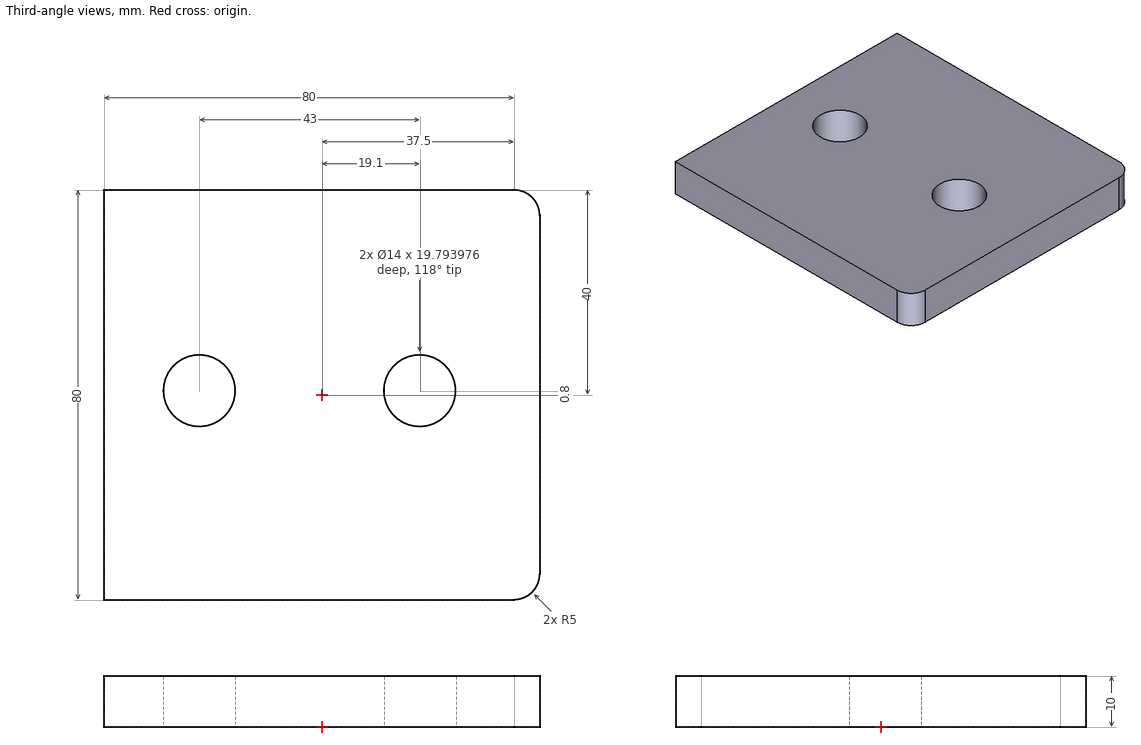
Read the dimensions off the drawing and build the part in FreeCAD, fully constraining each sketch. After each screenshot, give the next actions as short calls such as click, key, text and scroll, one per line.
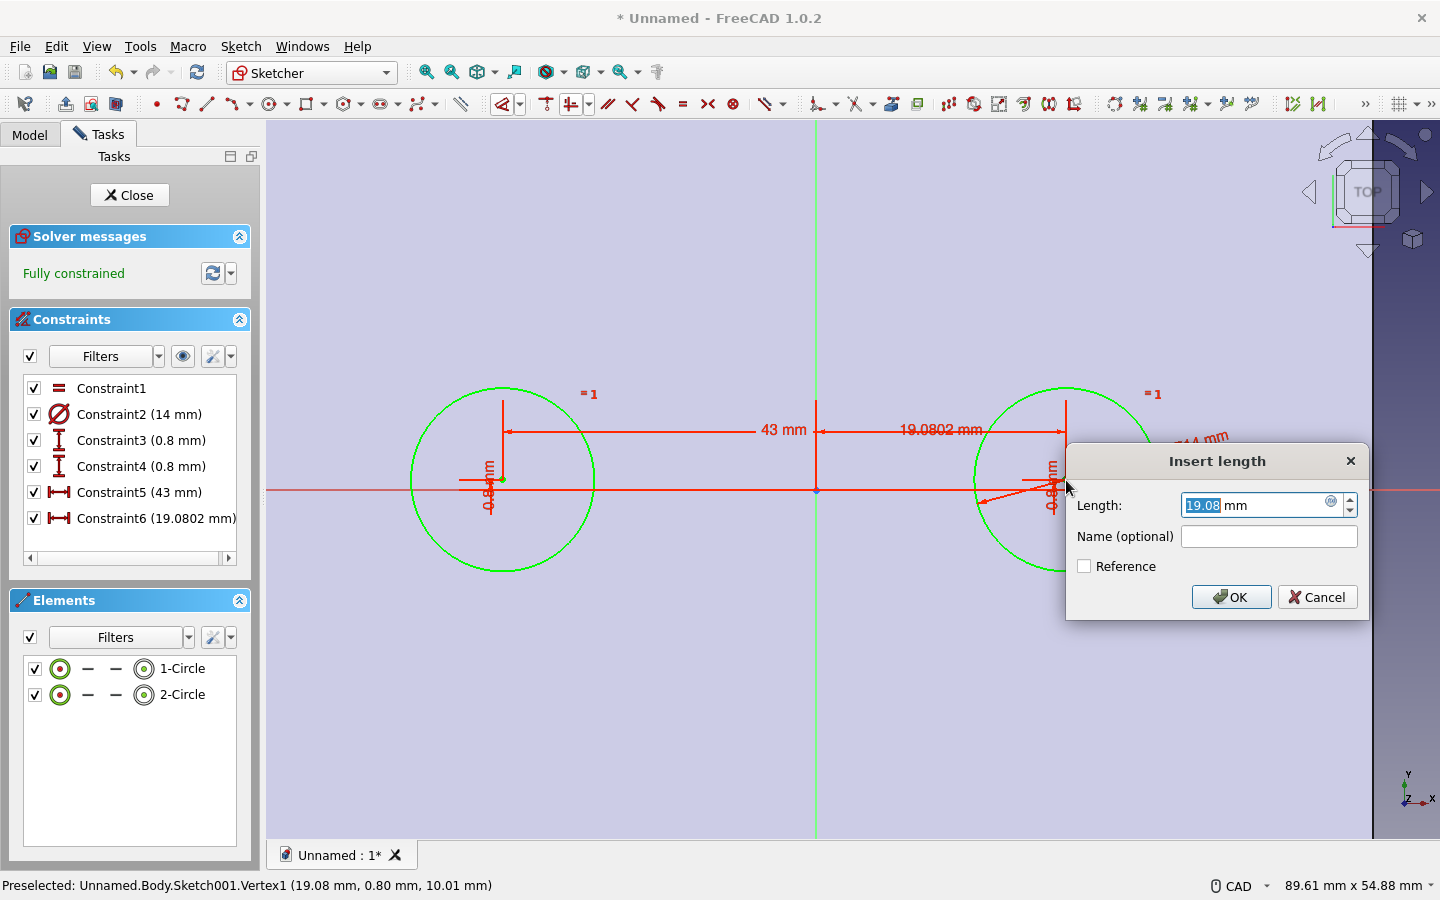
text(19.1)
key(Return)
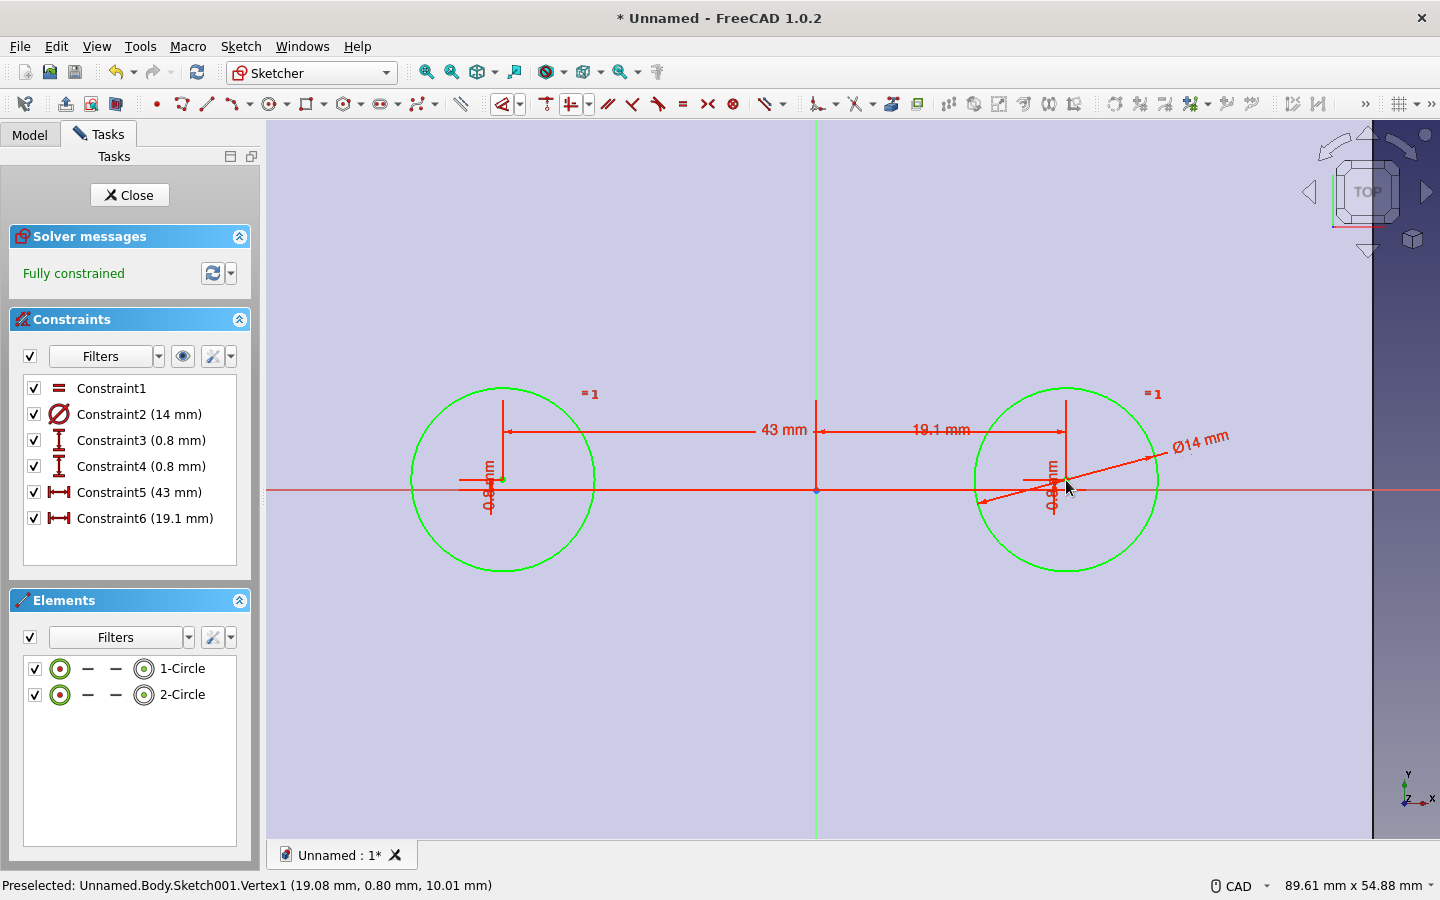
click(130, 195)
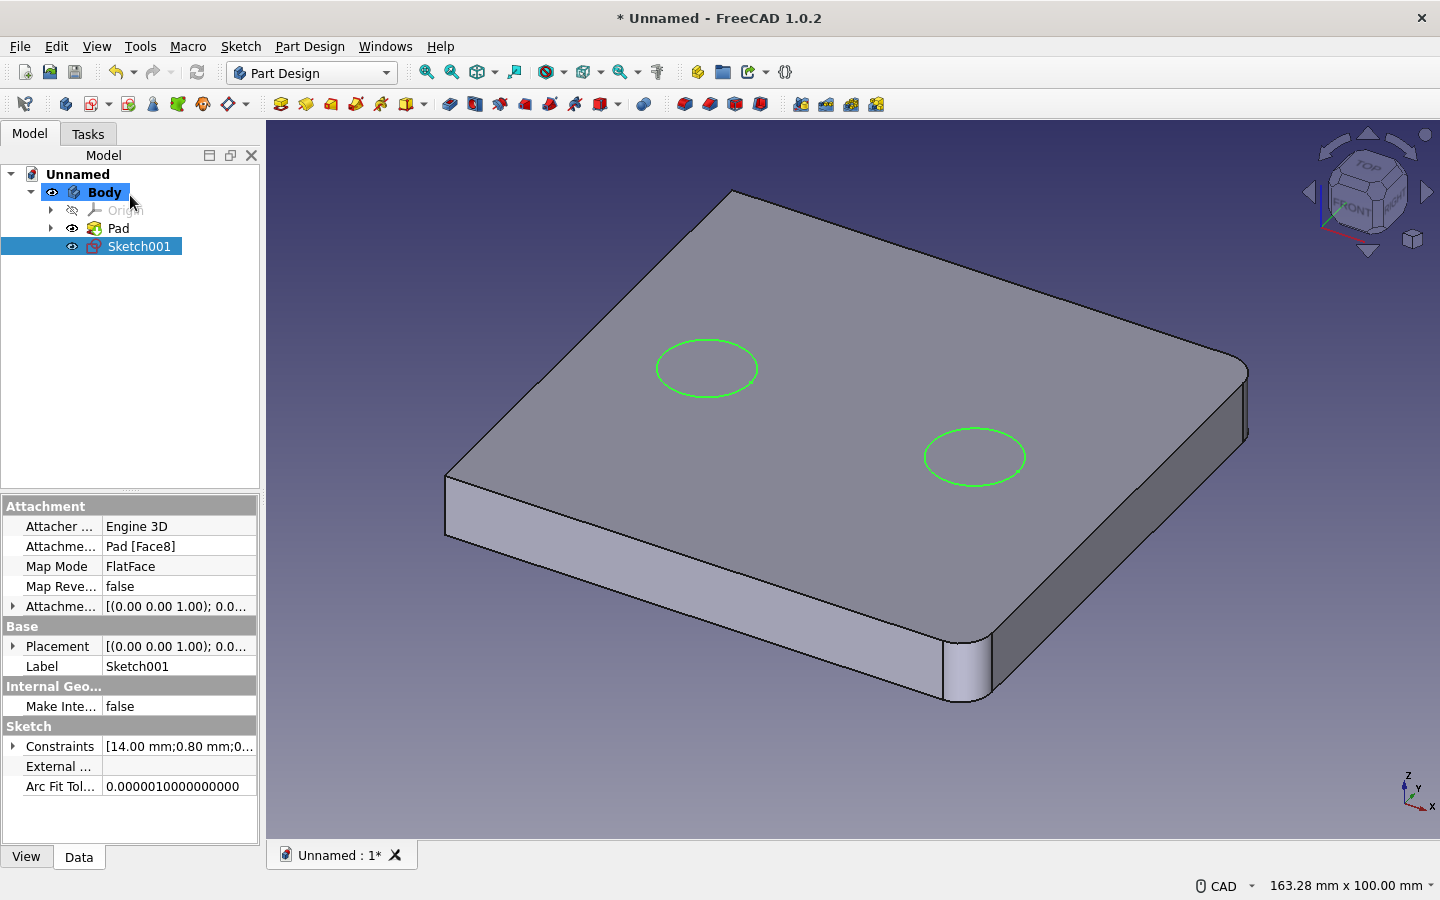
click(475, 104)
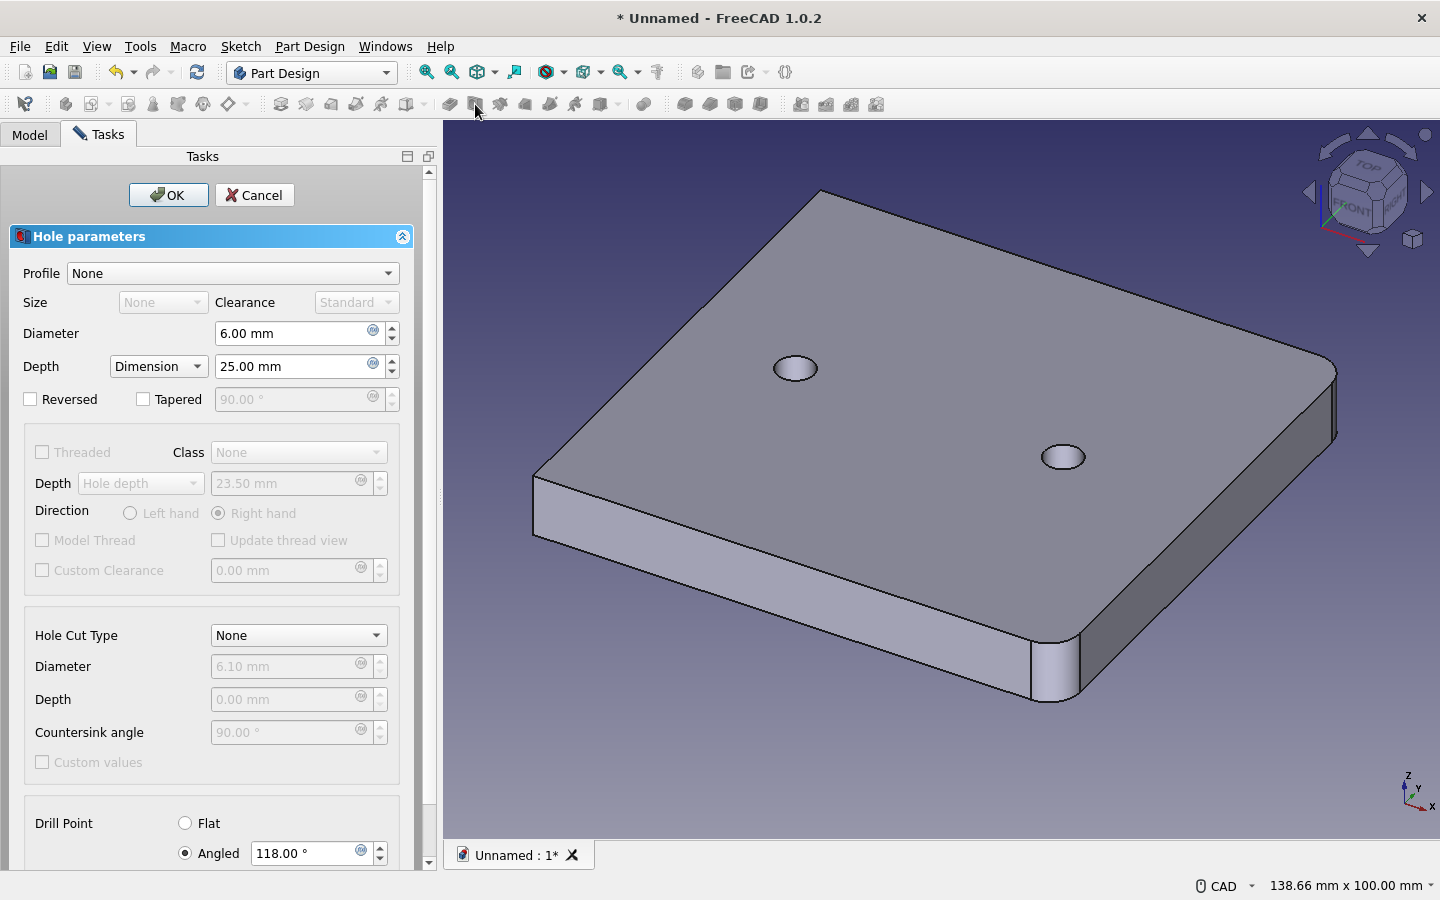
triple_click(300, 334)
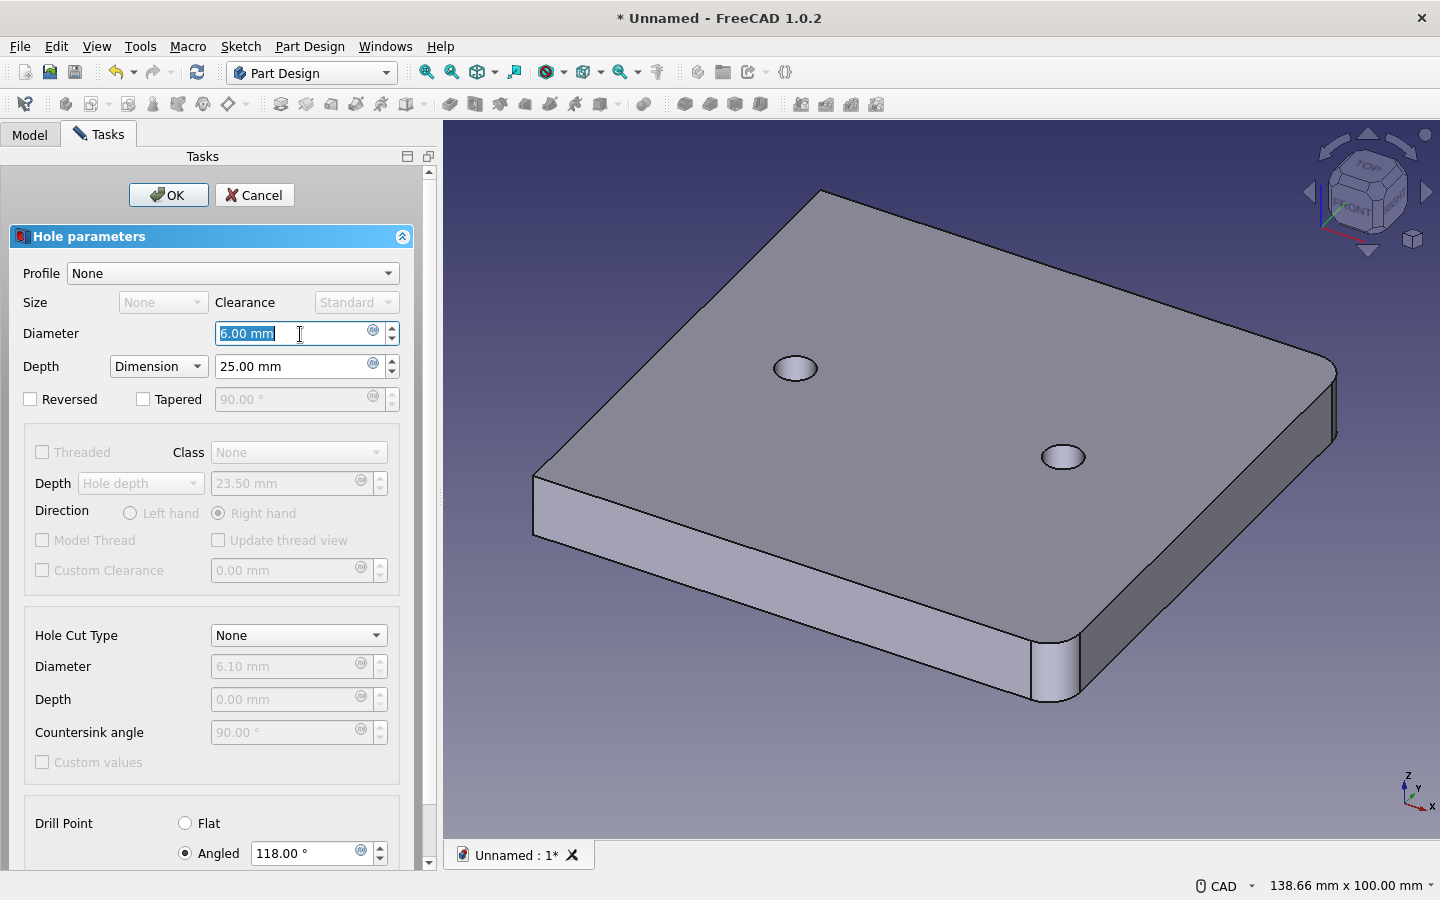
text(14)
key(Tab)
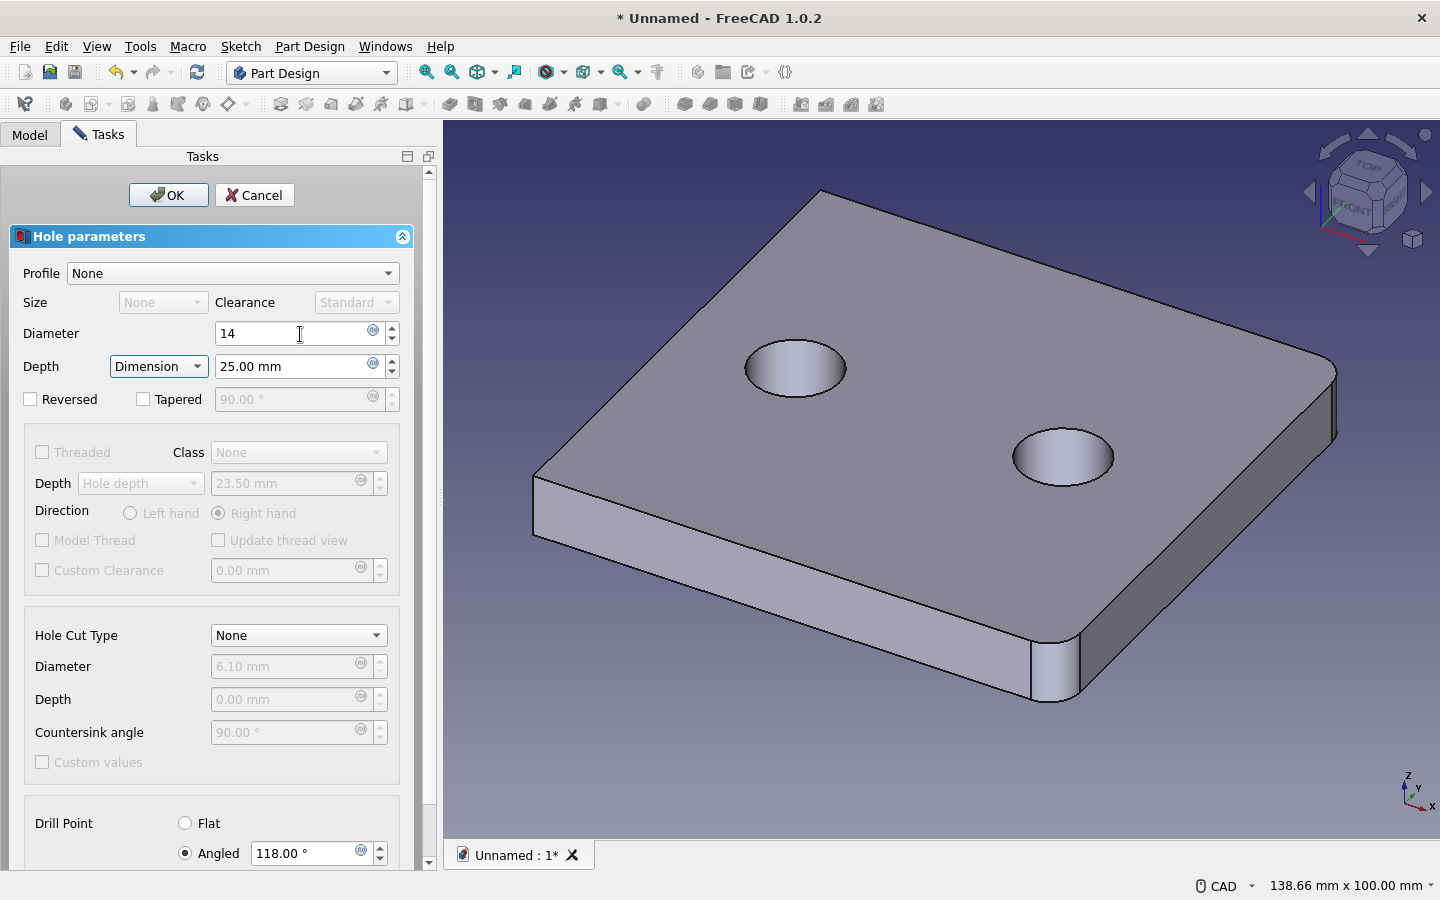
triple_click(300, 366)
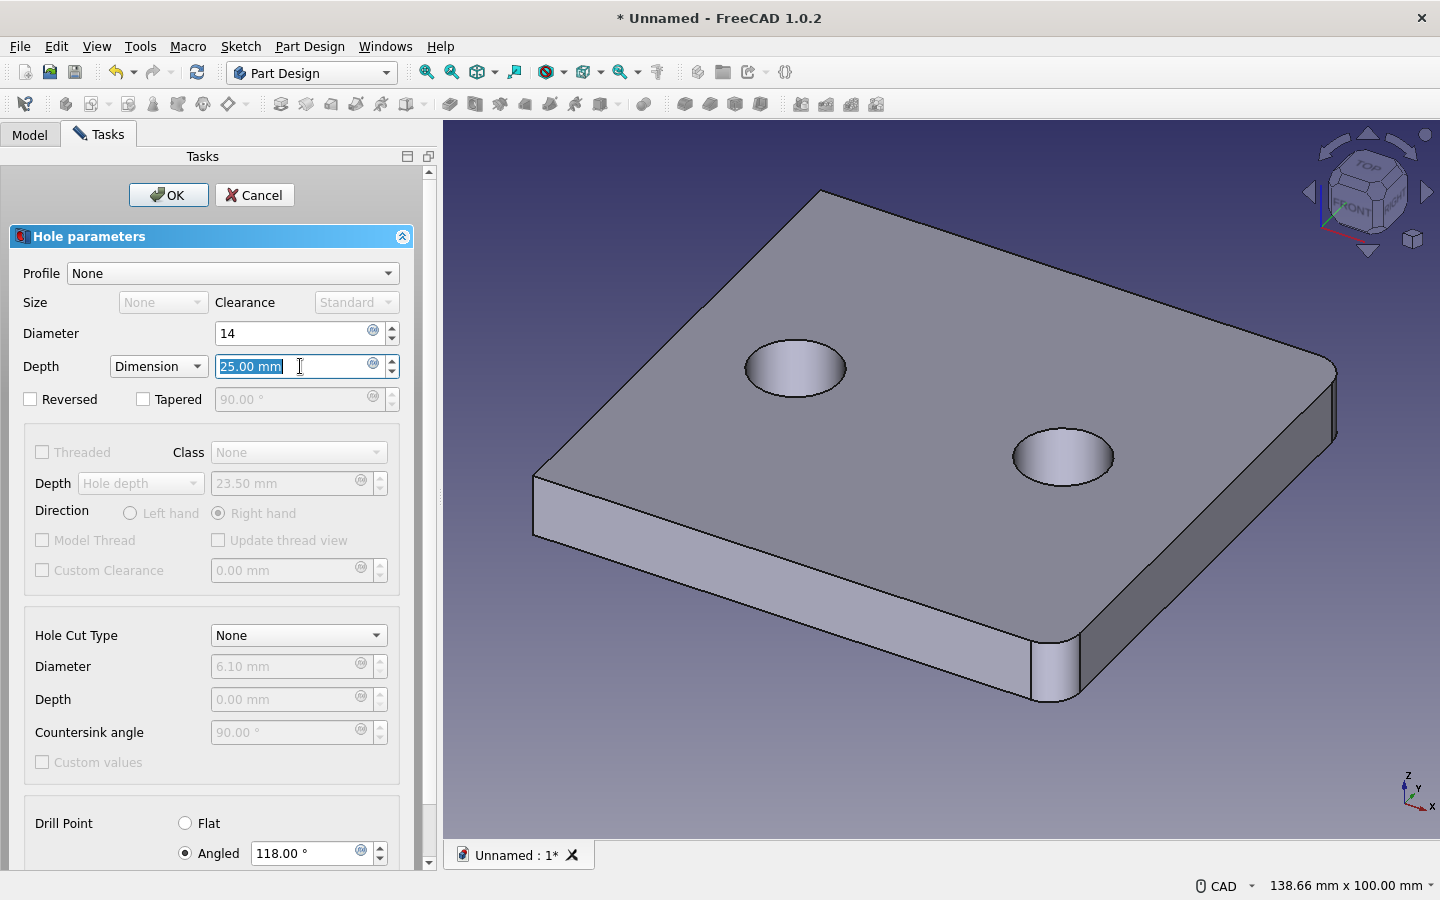
text(19.793976)
key(Tab)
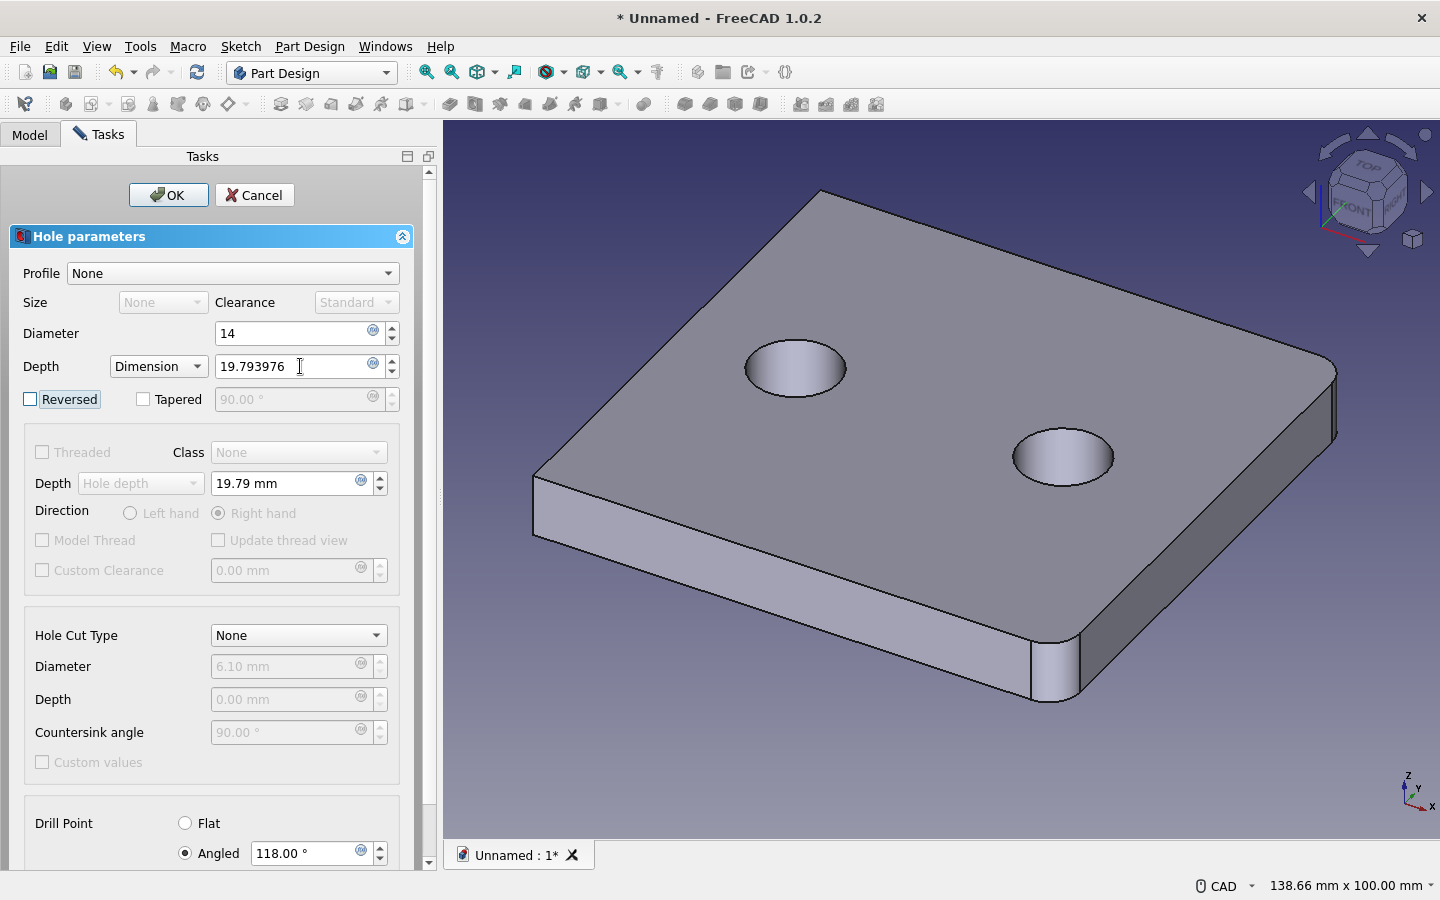
click(169, 195)